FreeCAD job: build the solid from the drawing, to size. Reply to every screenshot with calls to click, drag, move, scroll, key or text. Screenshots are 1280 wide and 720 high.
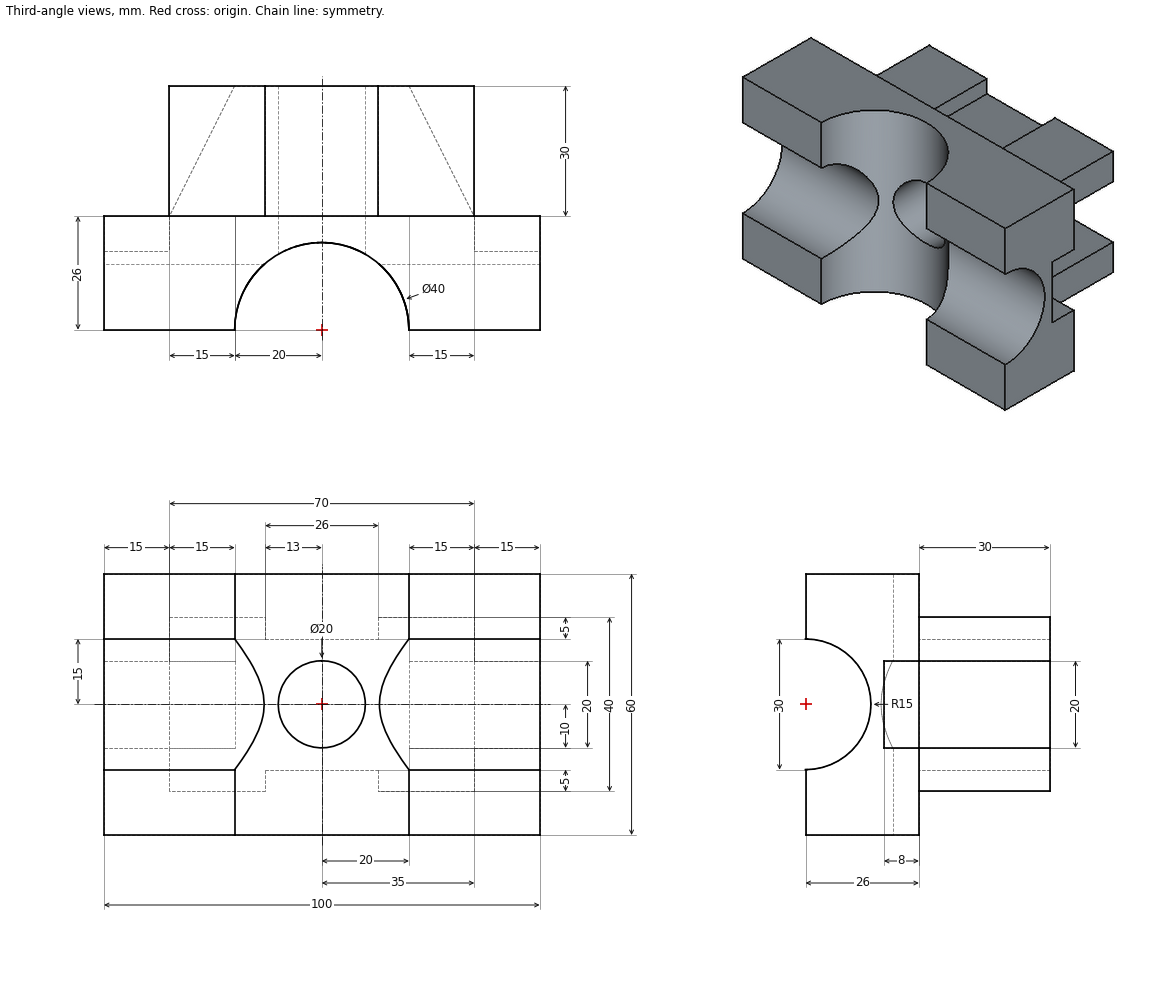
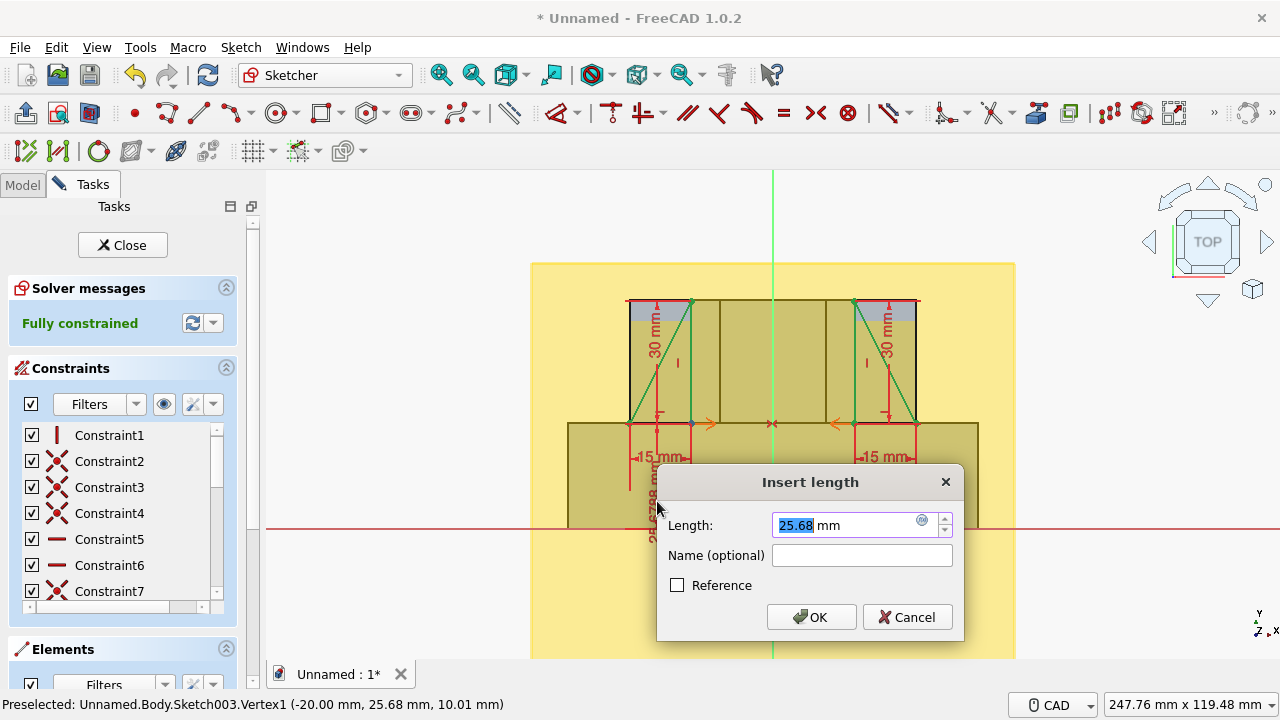
text(26)
key(Return)
key(Escape)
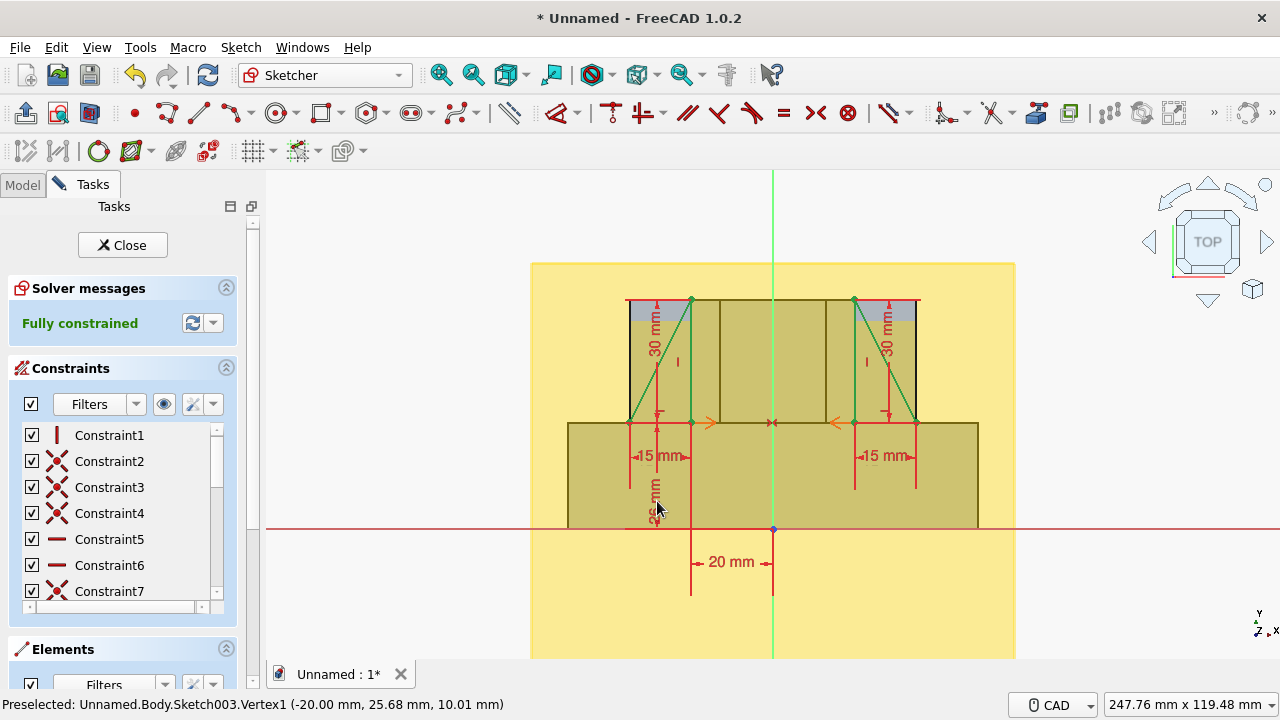
click(123, 245)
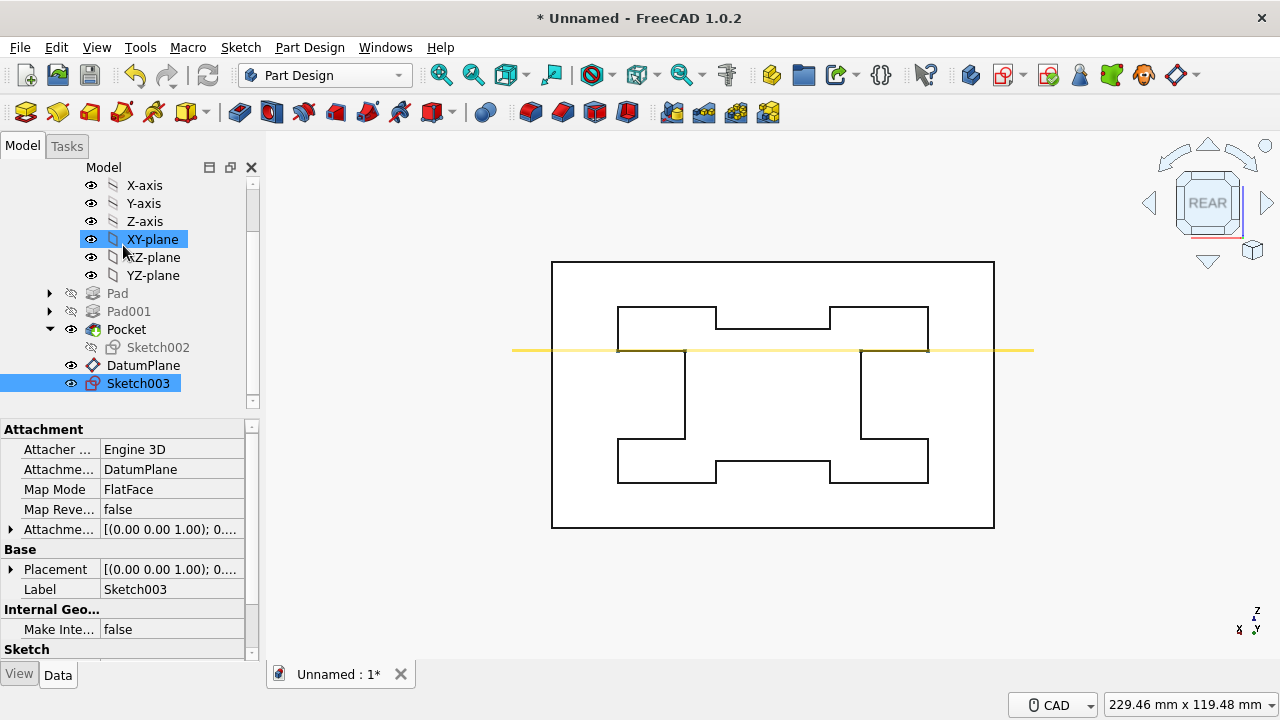
click(26, 112)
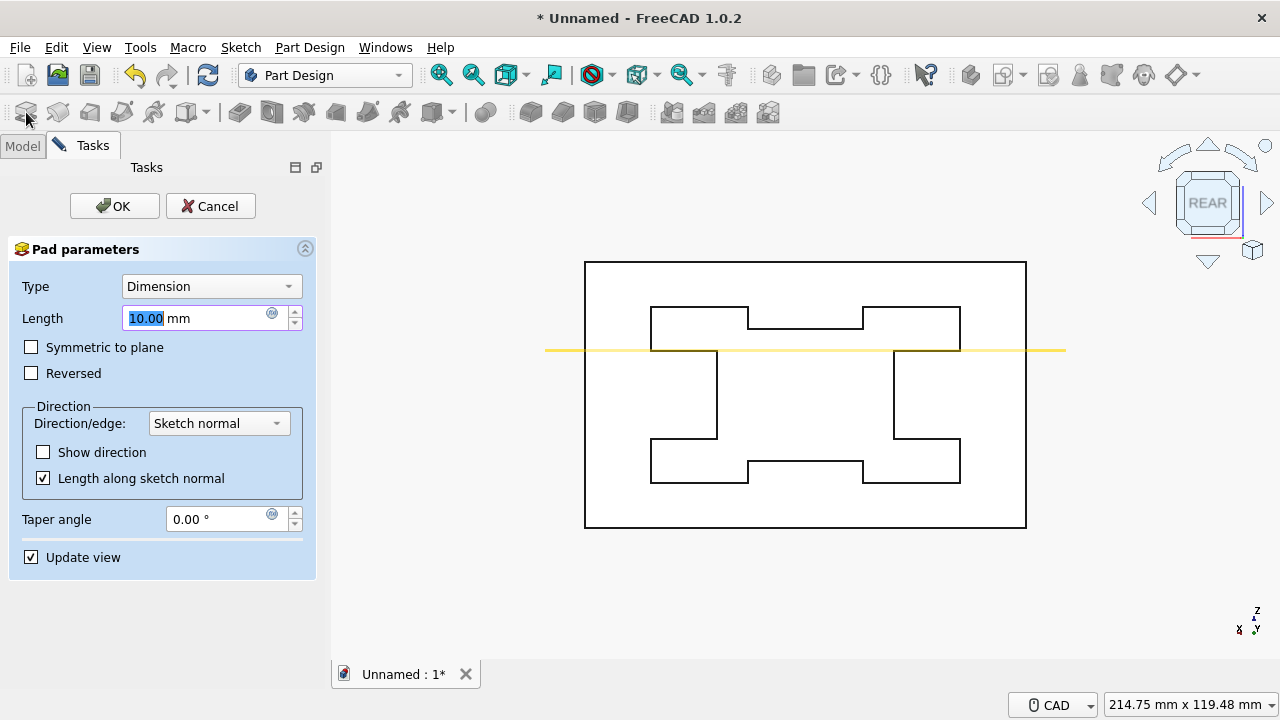
text(20)
key(Tab)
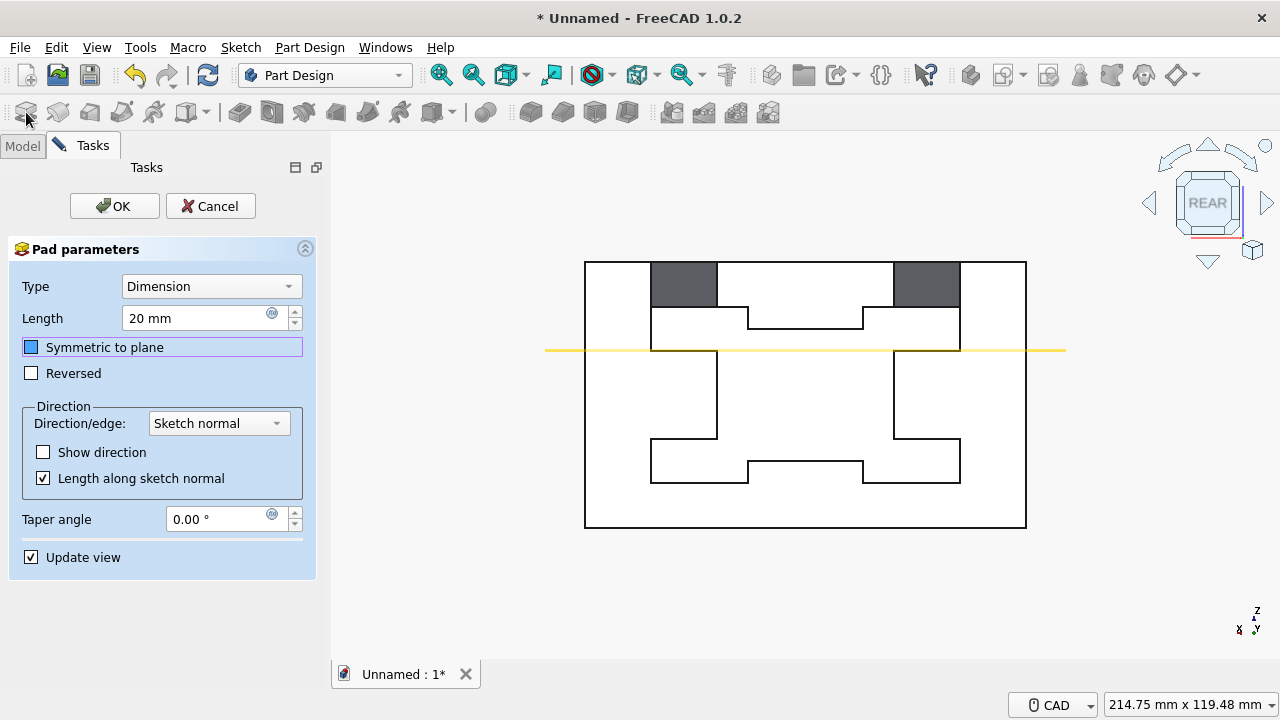
click(30, 373)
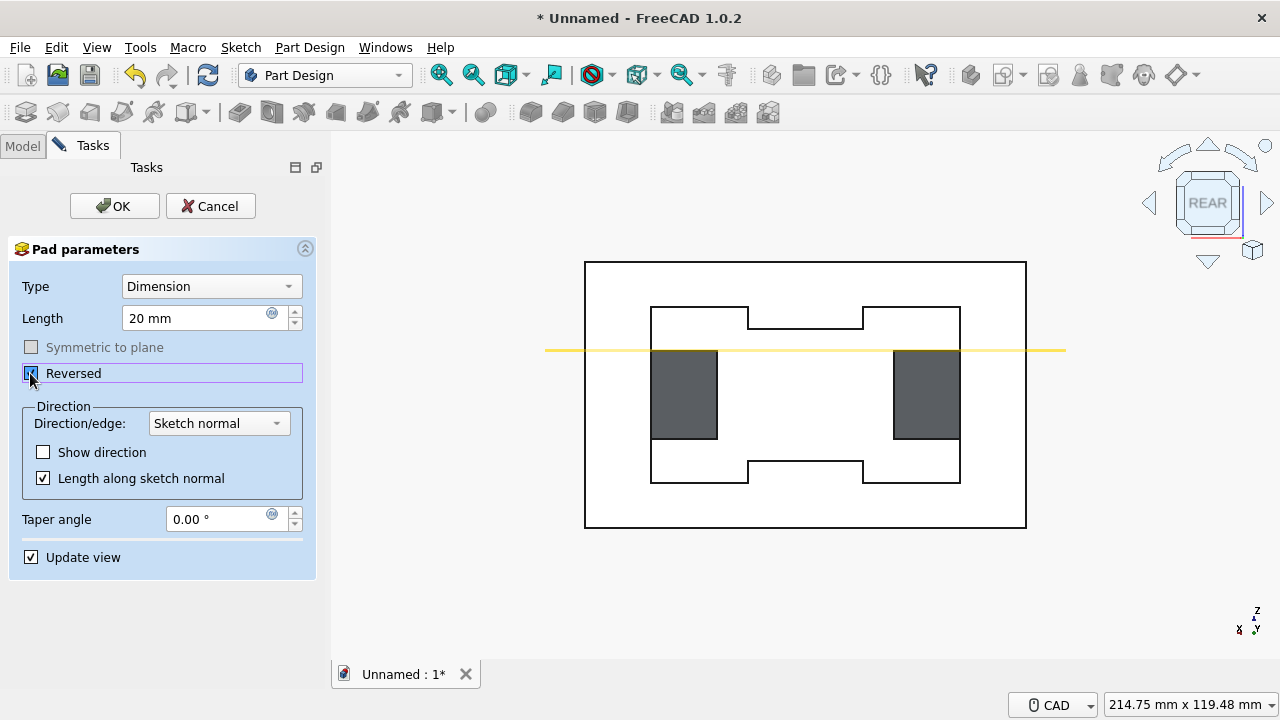
click(115, 206)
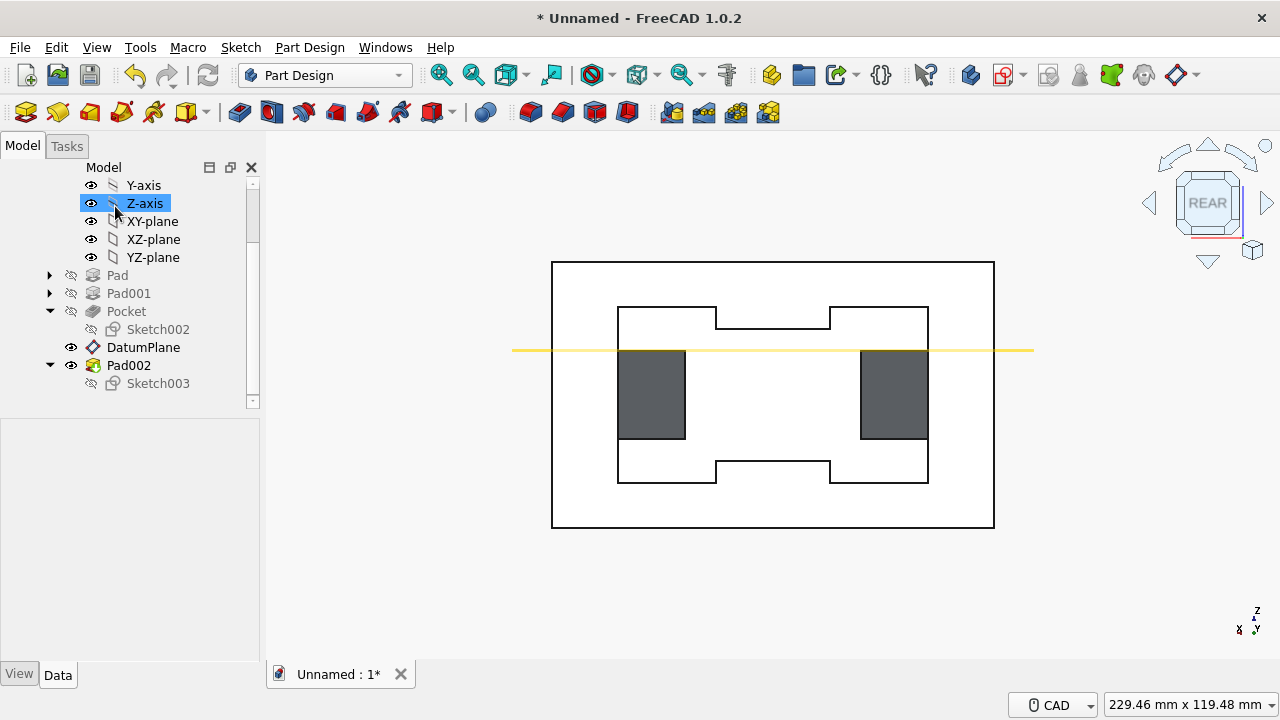
click(116, 347)
key(space)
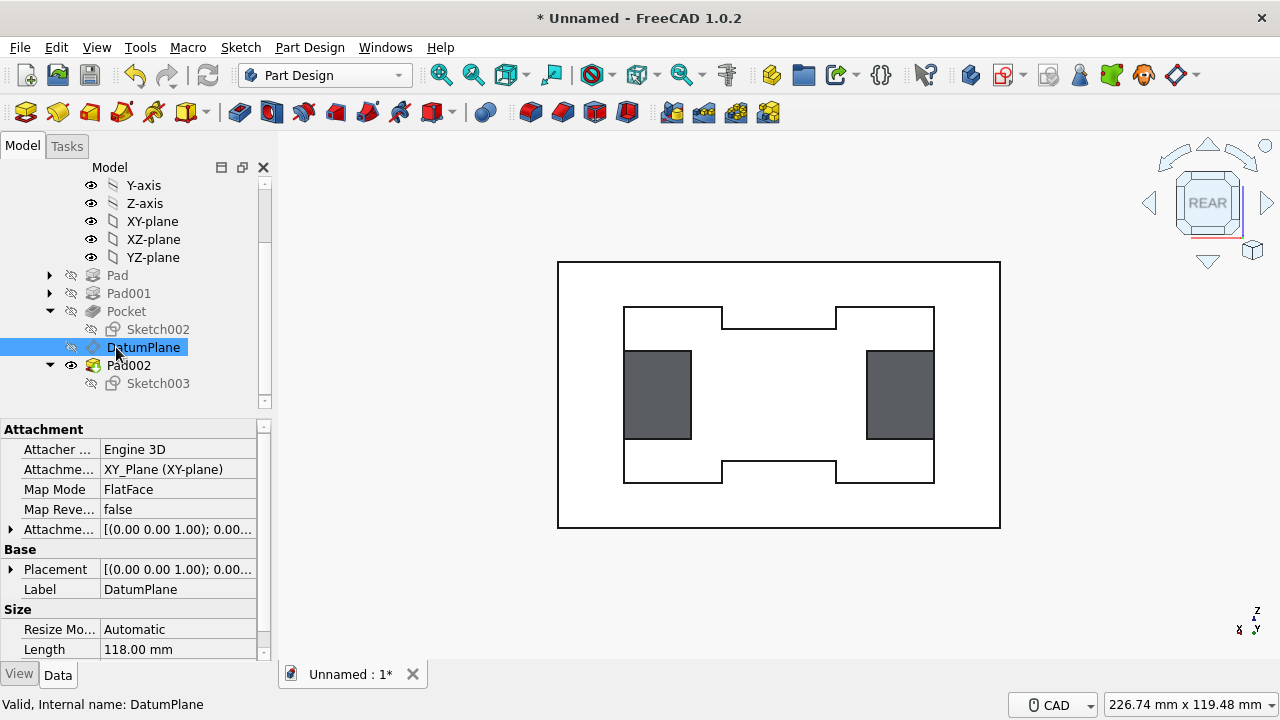
click(779, 394)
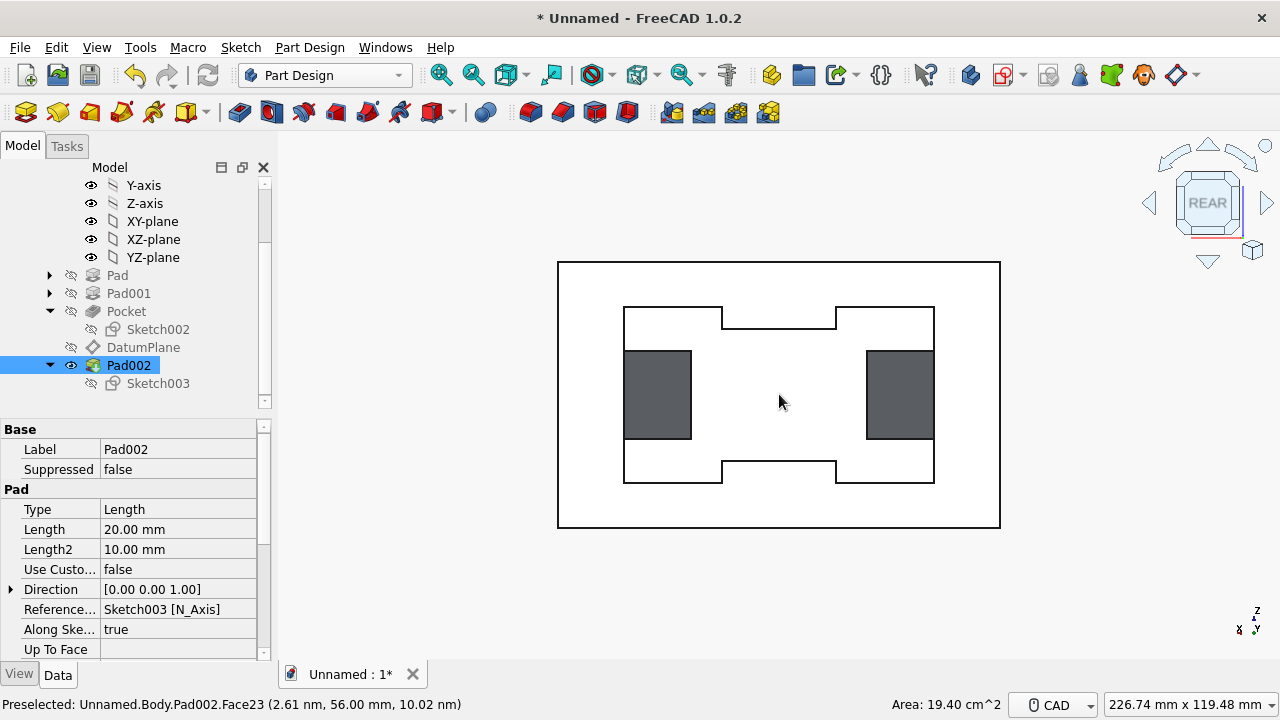
click(1004, 76)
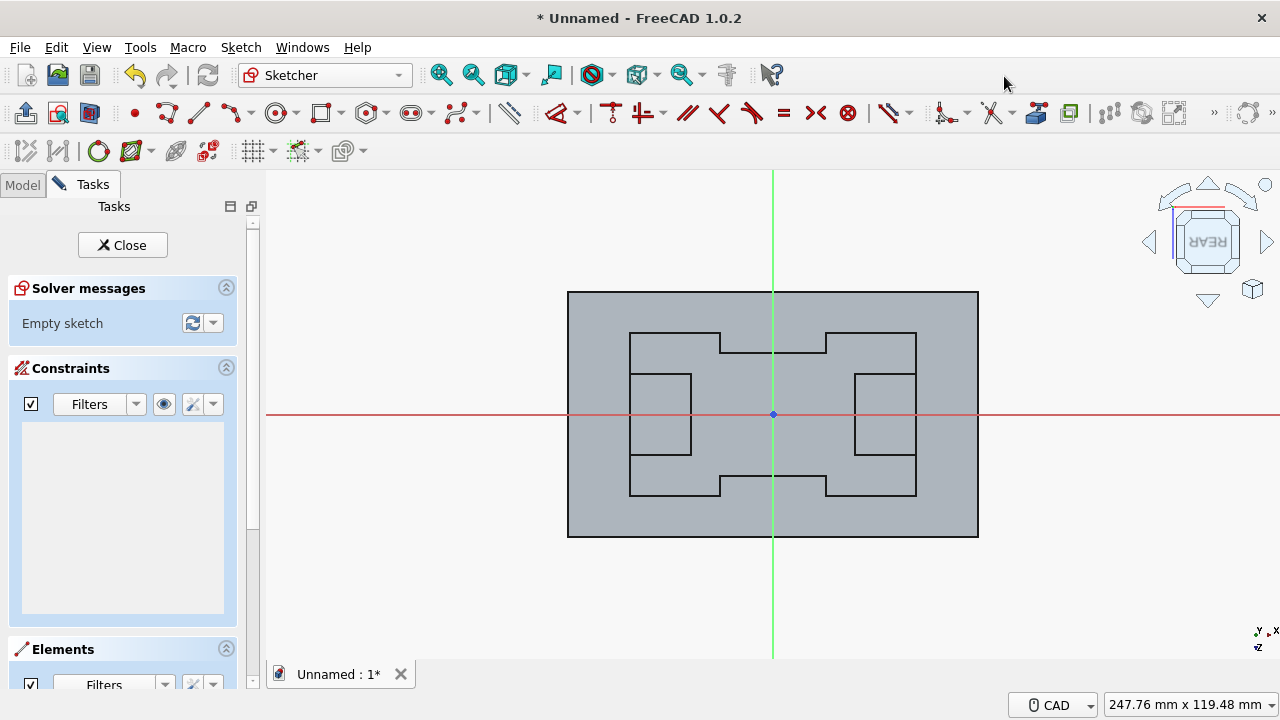
scroll(795, 414, up, 7)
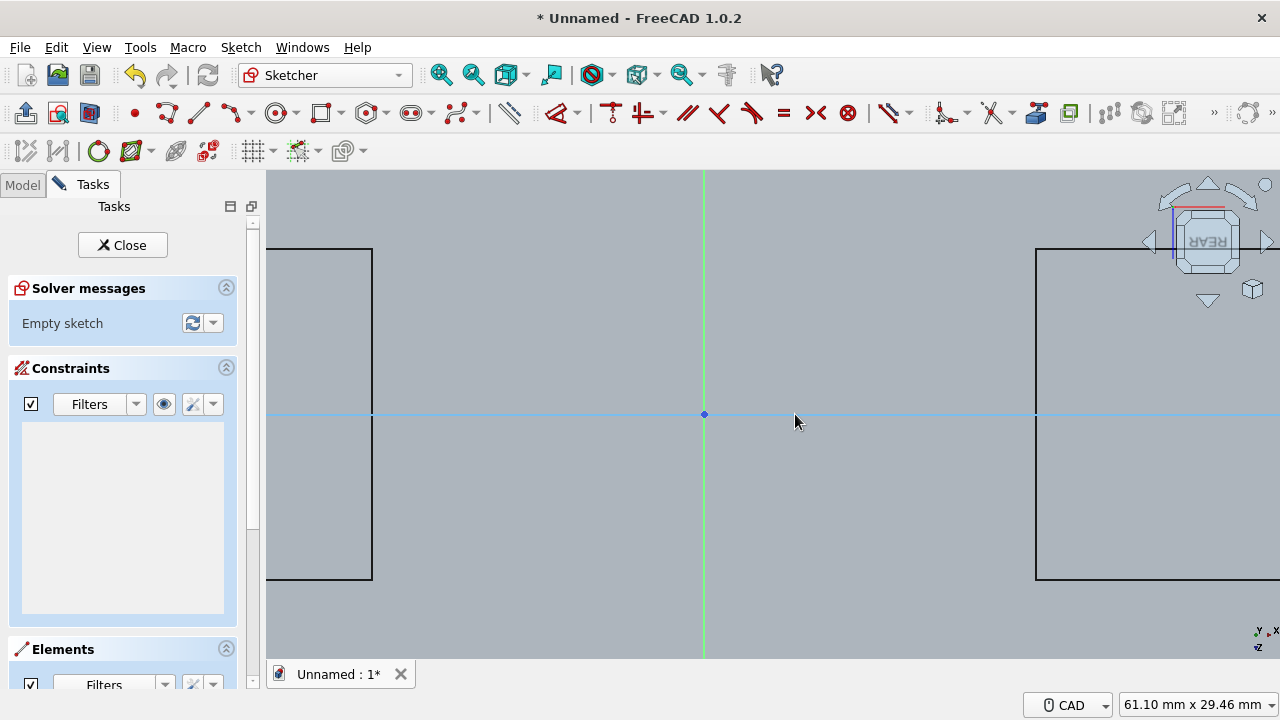
key(g)
key(c)